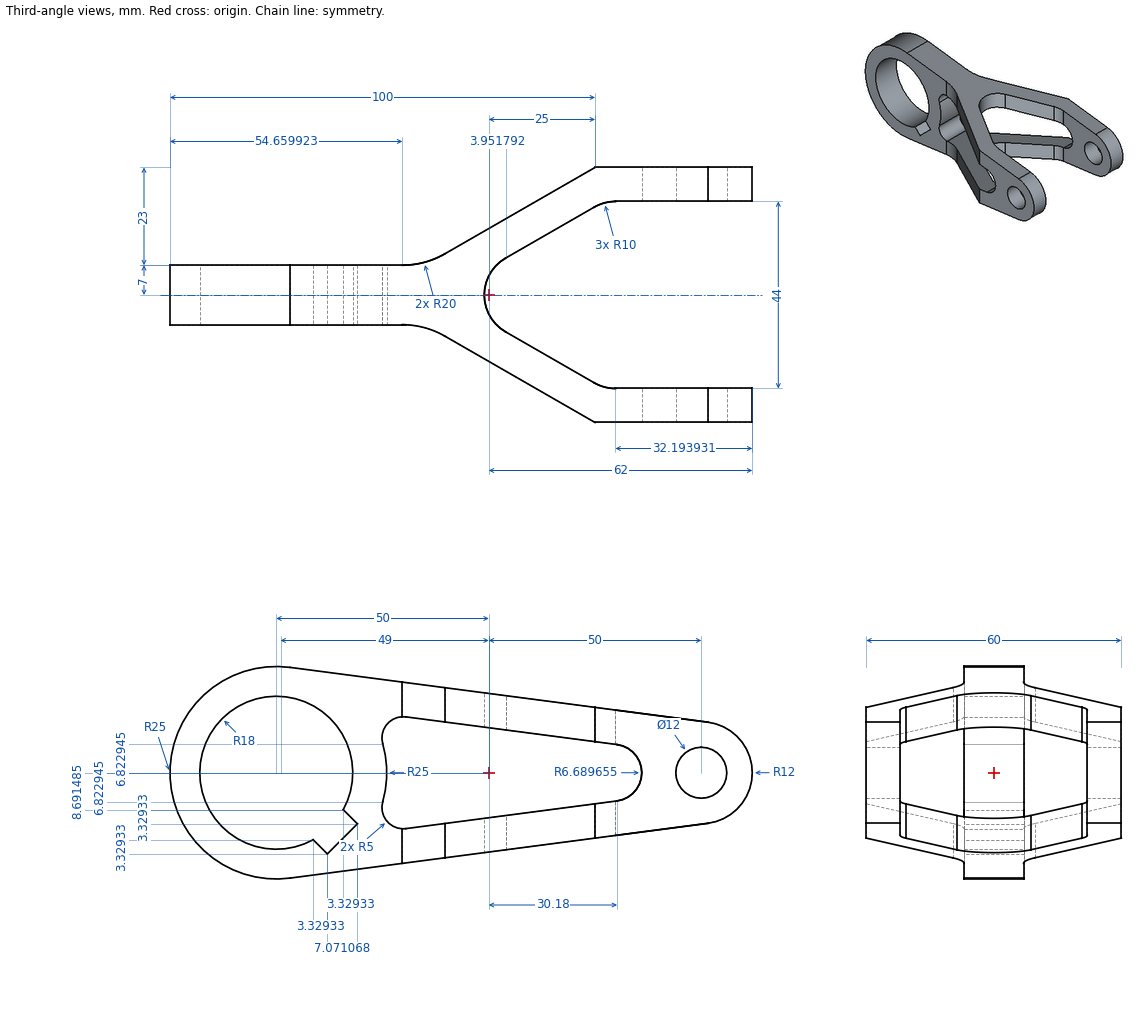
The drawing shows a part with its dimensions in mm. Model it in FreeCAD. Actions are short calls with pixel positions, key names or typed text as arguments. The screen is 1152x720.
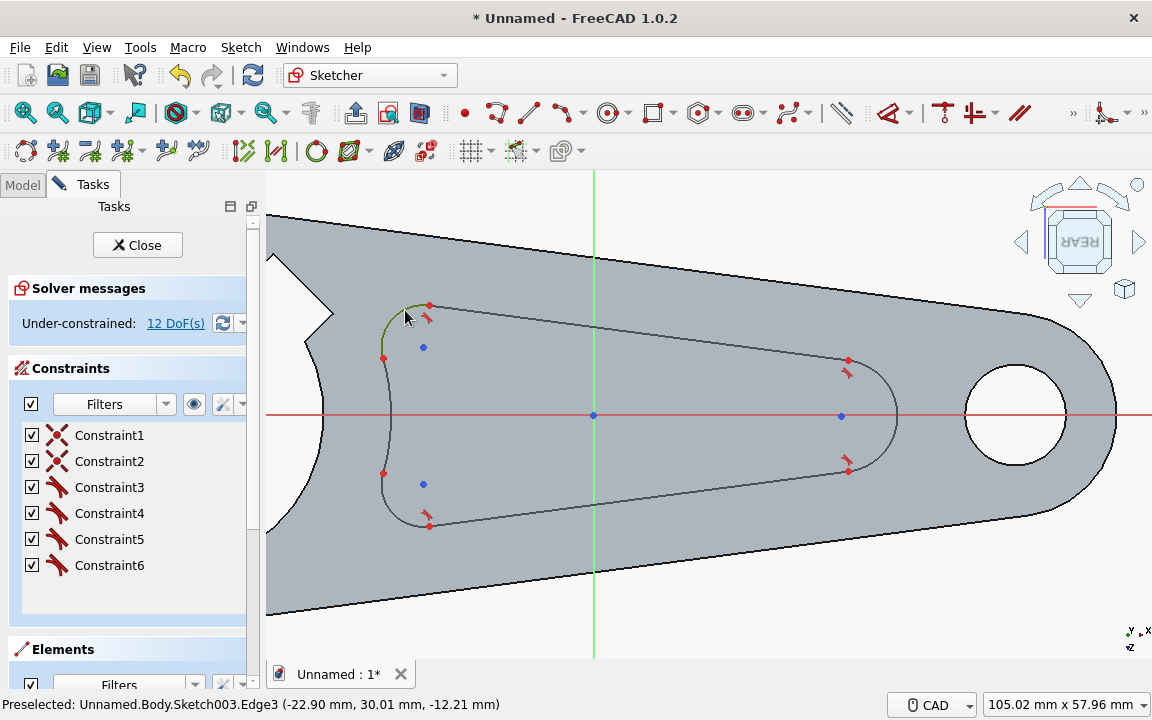
click(390, 439)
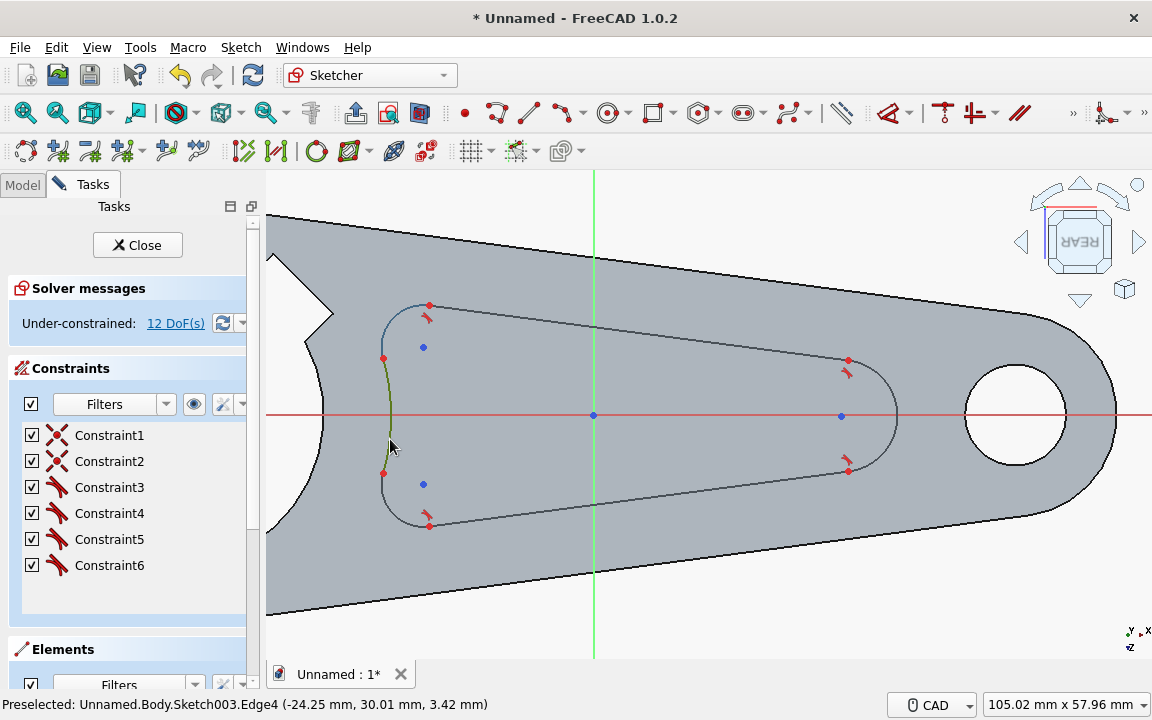
key(t)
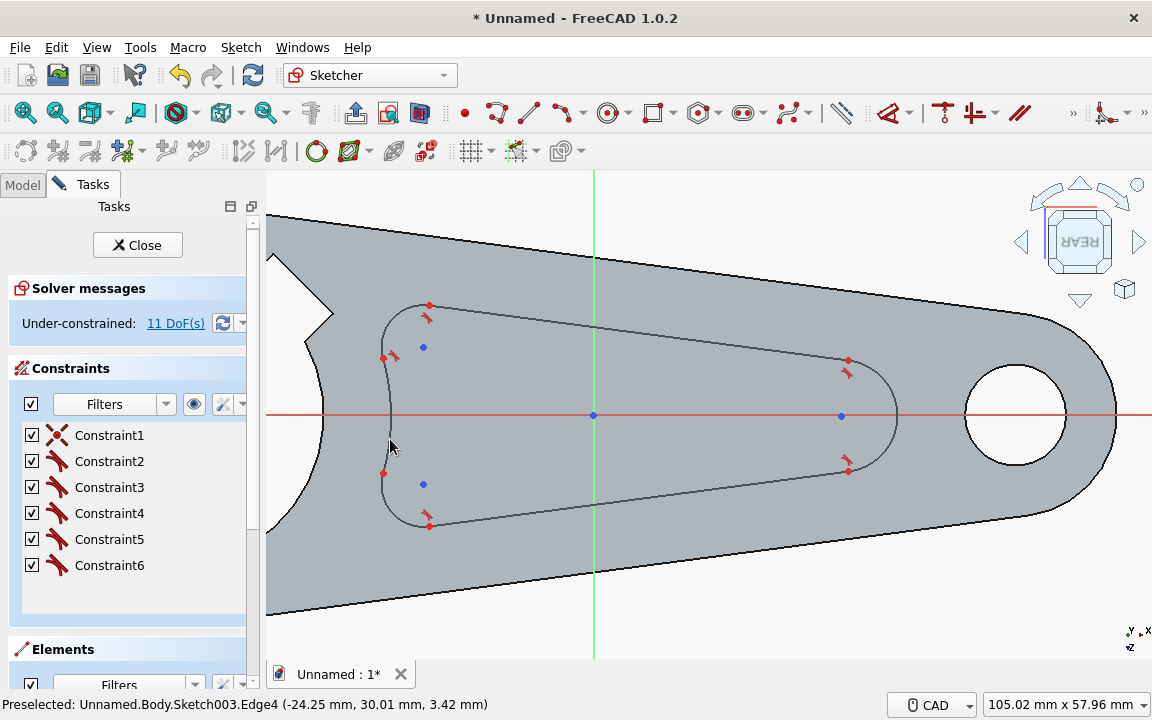
click(390, 439)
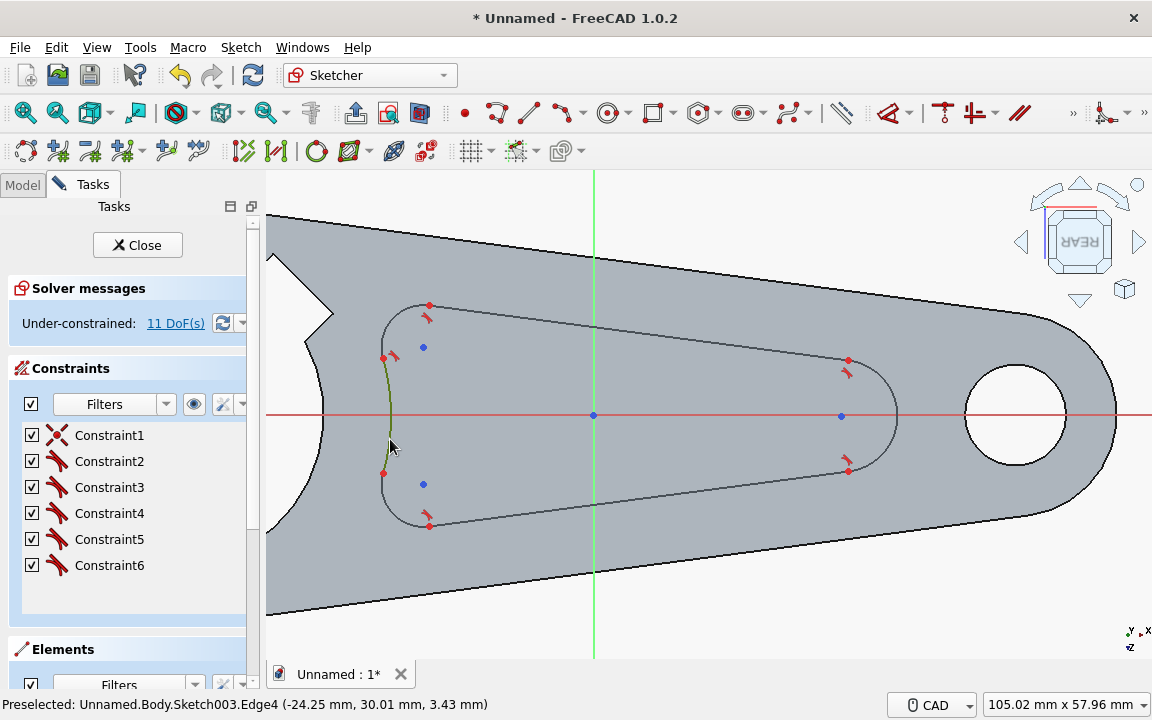
click(384, 498)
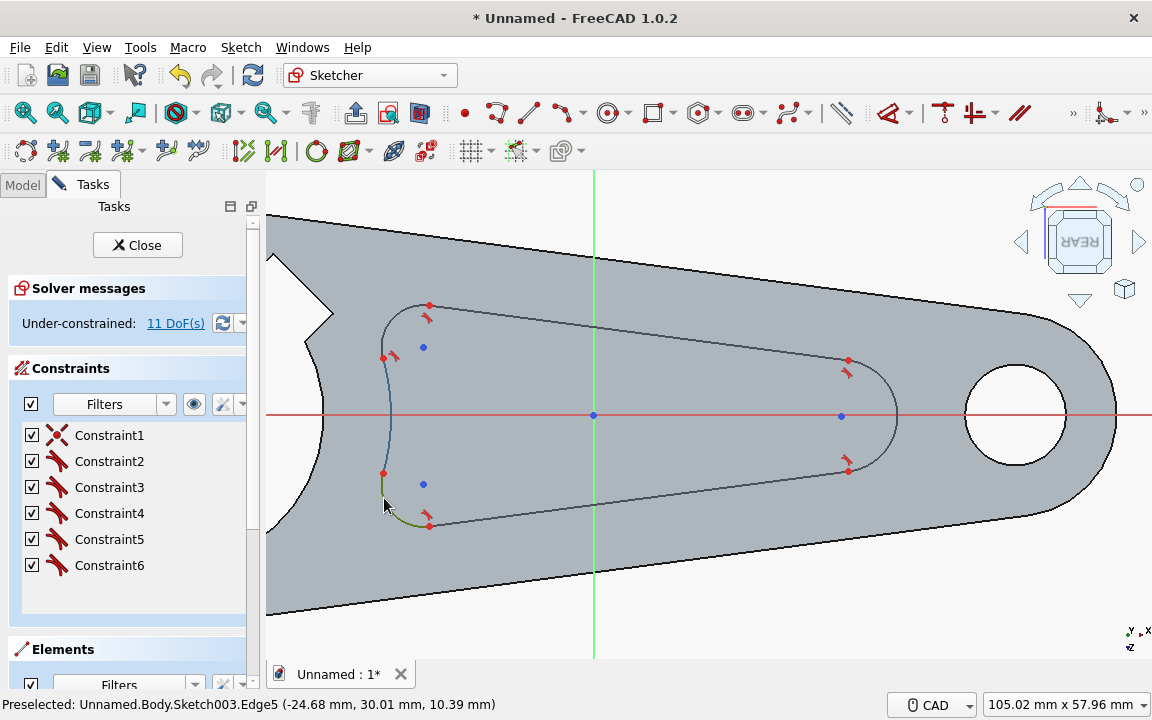
key(t)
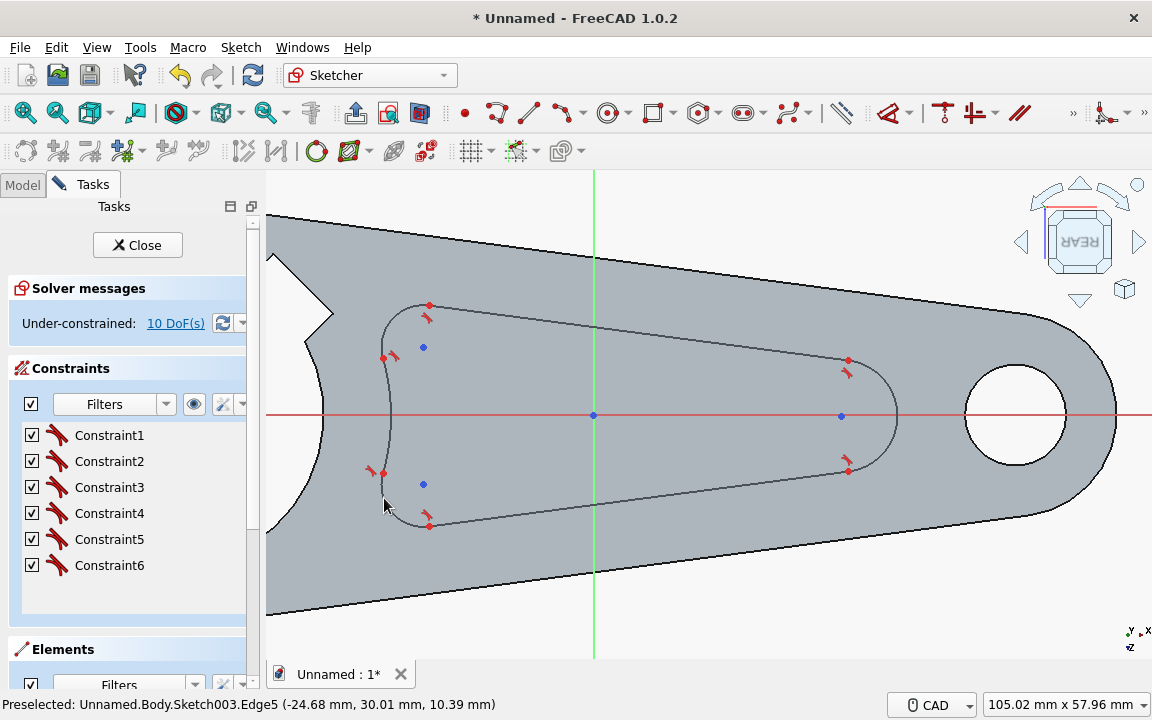
click(405, 310)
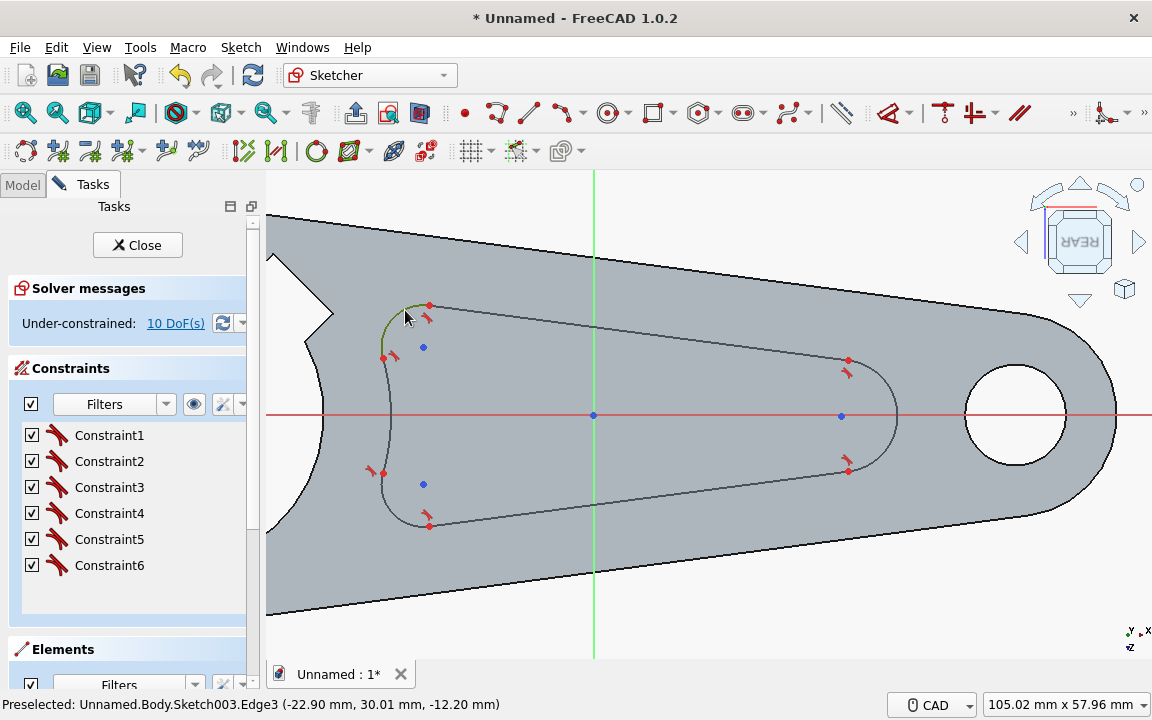
click(384, 498)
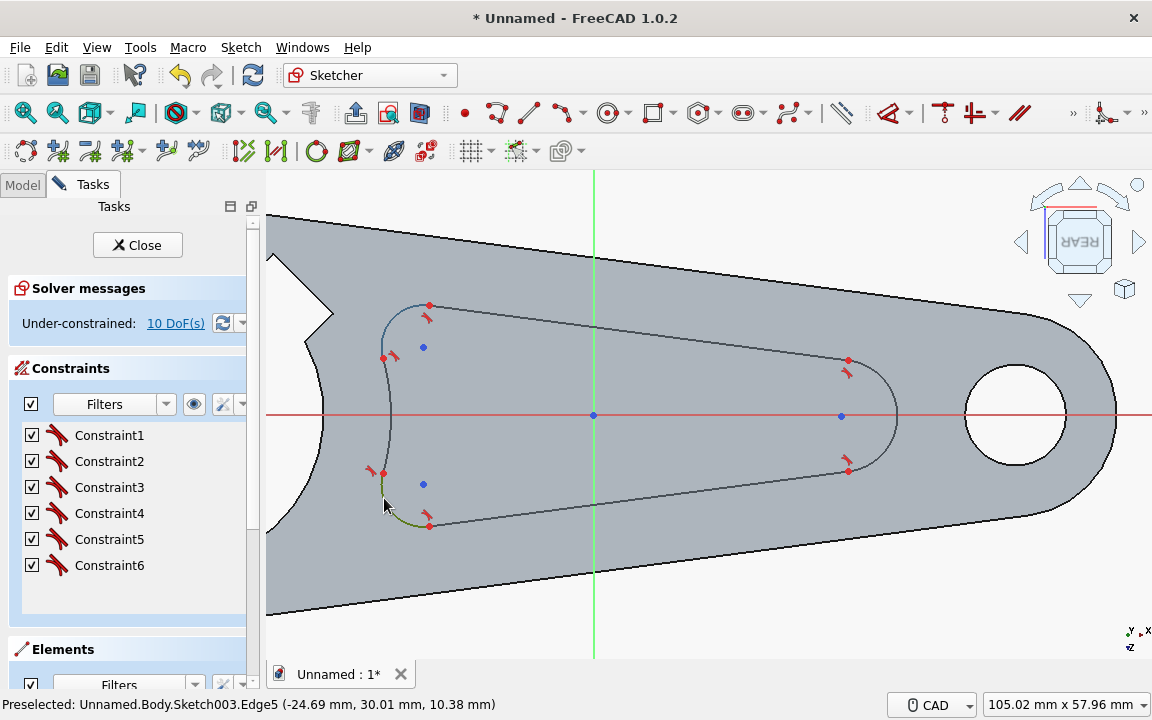
key(e)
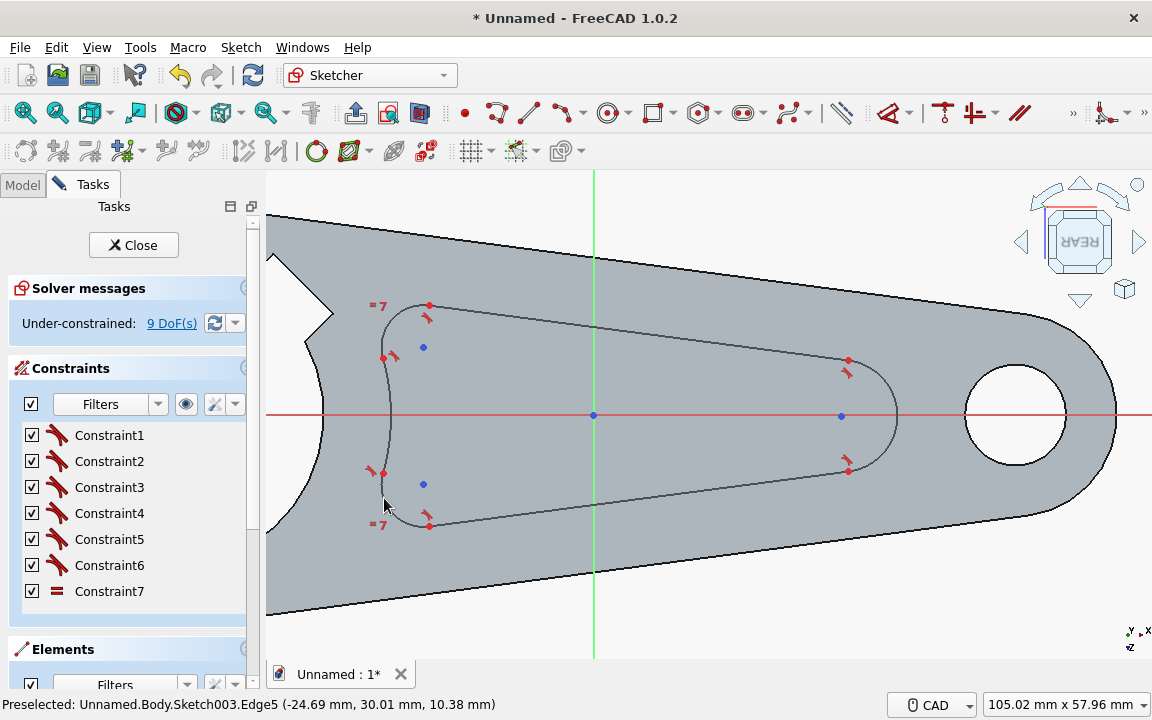
scroll(849, 413, down, 2)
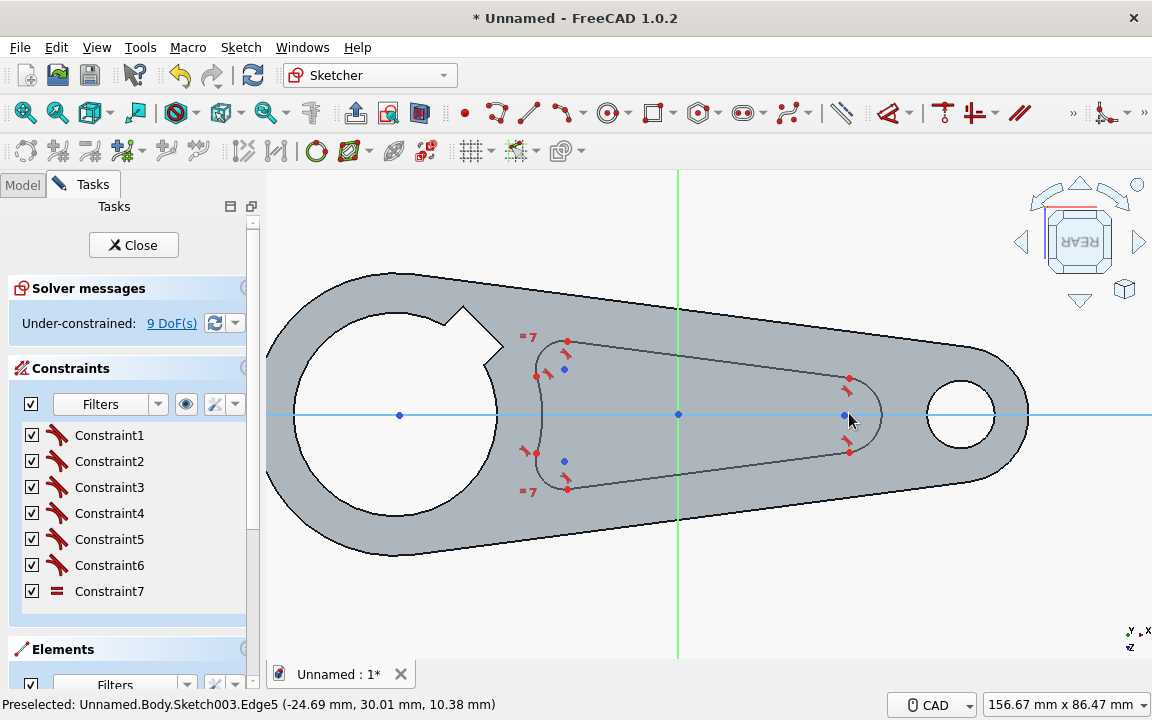
click(400, 415)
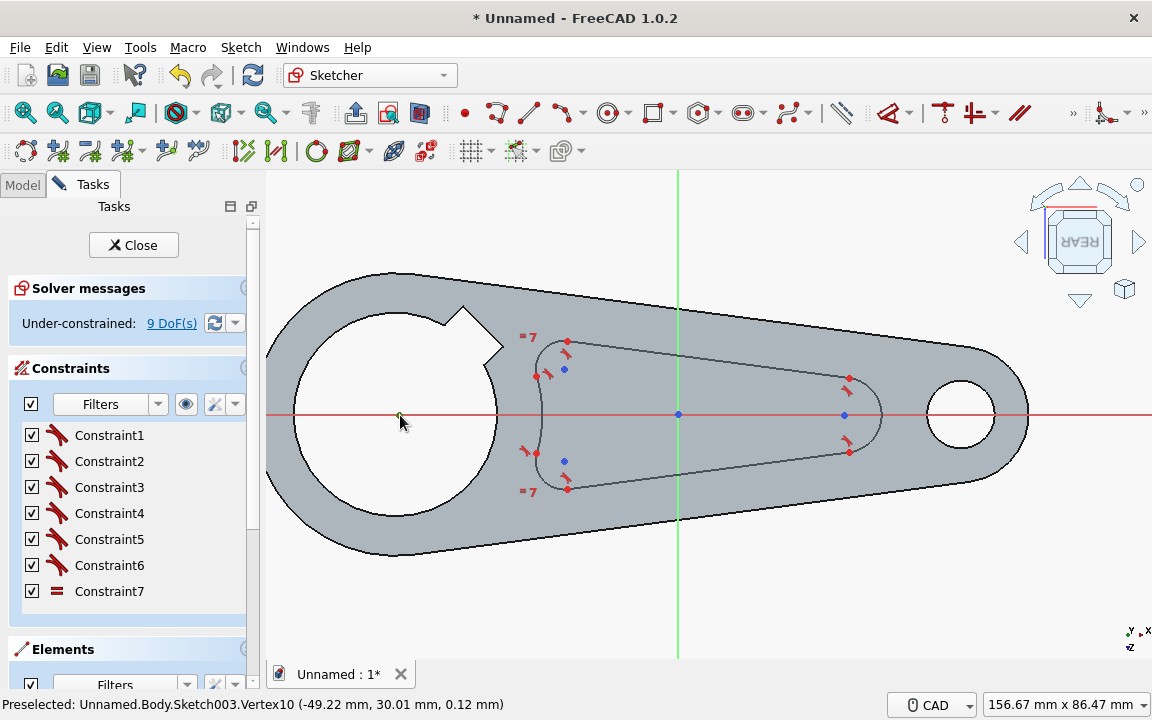
click(344, 415)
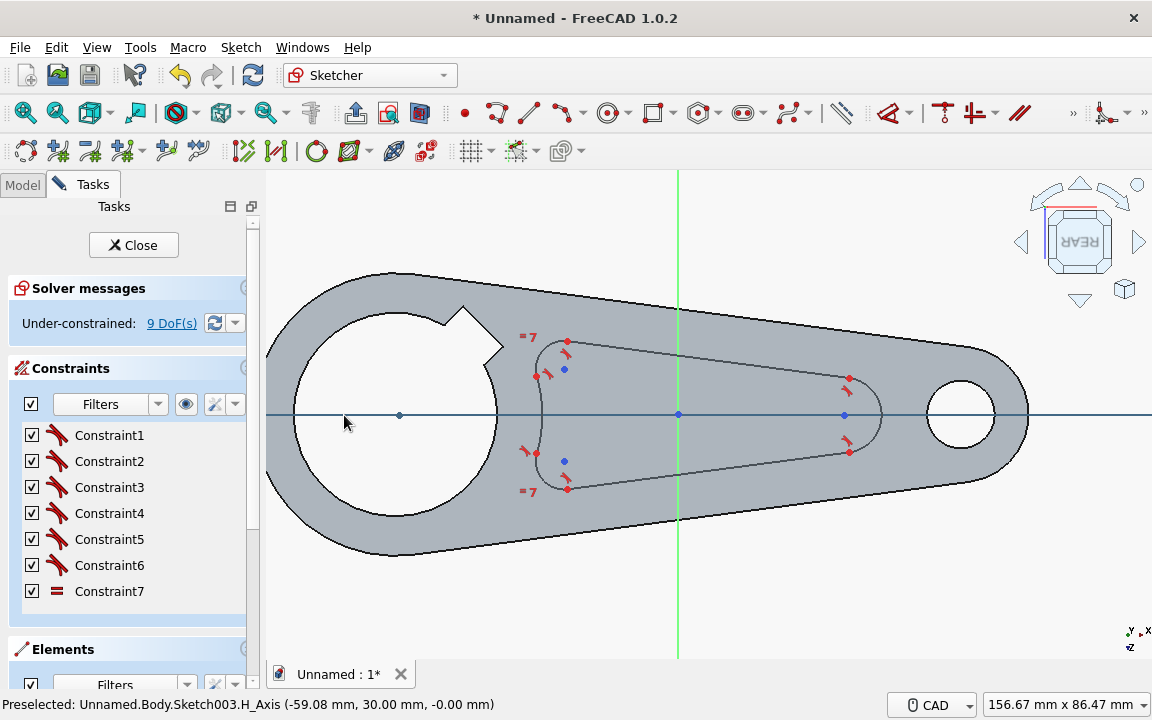
key(c)